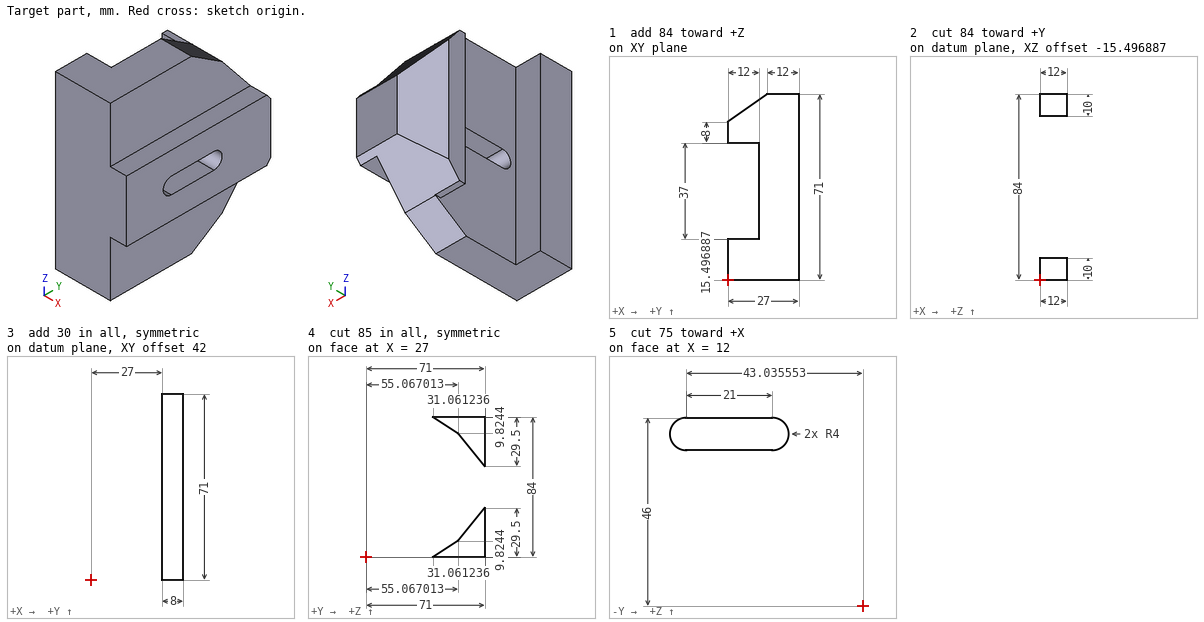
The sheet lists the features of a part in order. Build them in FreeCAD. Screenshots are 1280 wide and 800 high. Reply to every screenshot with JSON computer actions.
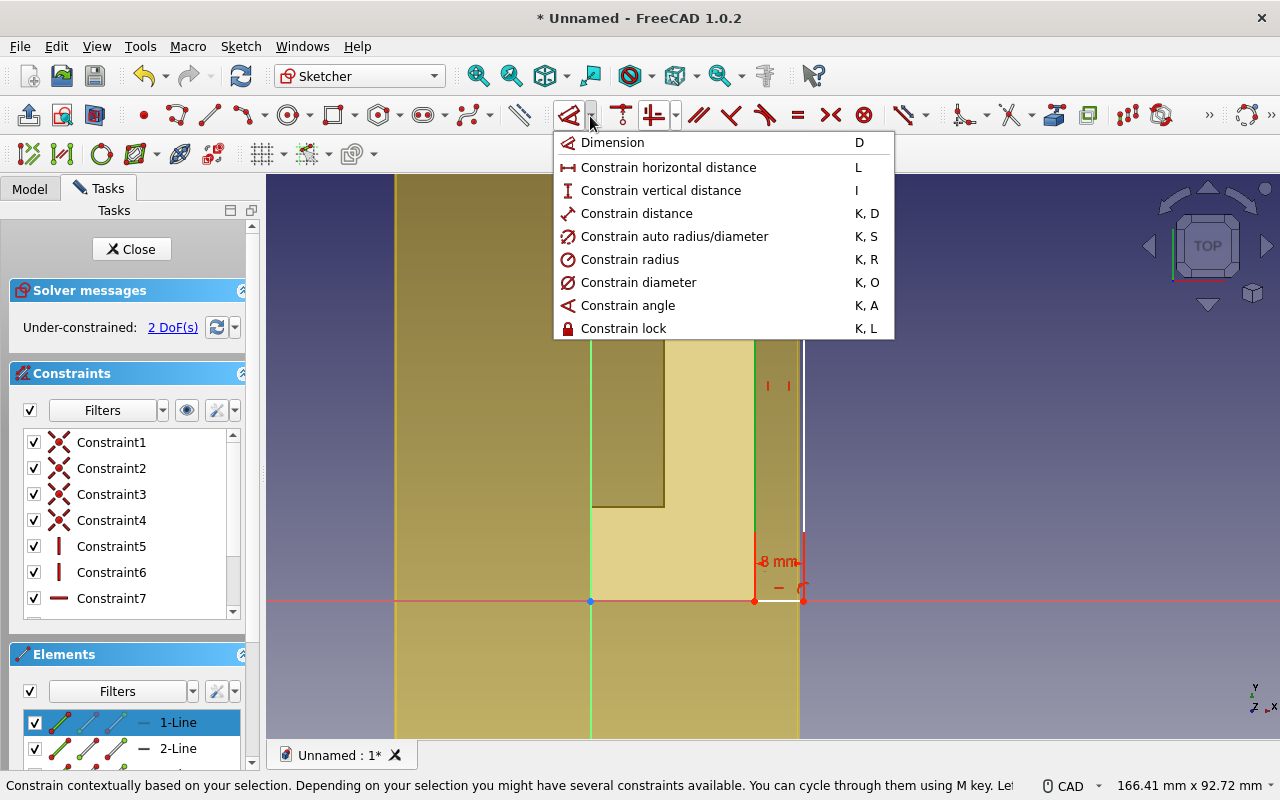
{"action": "left_click", "coordinate": [724, 190]}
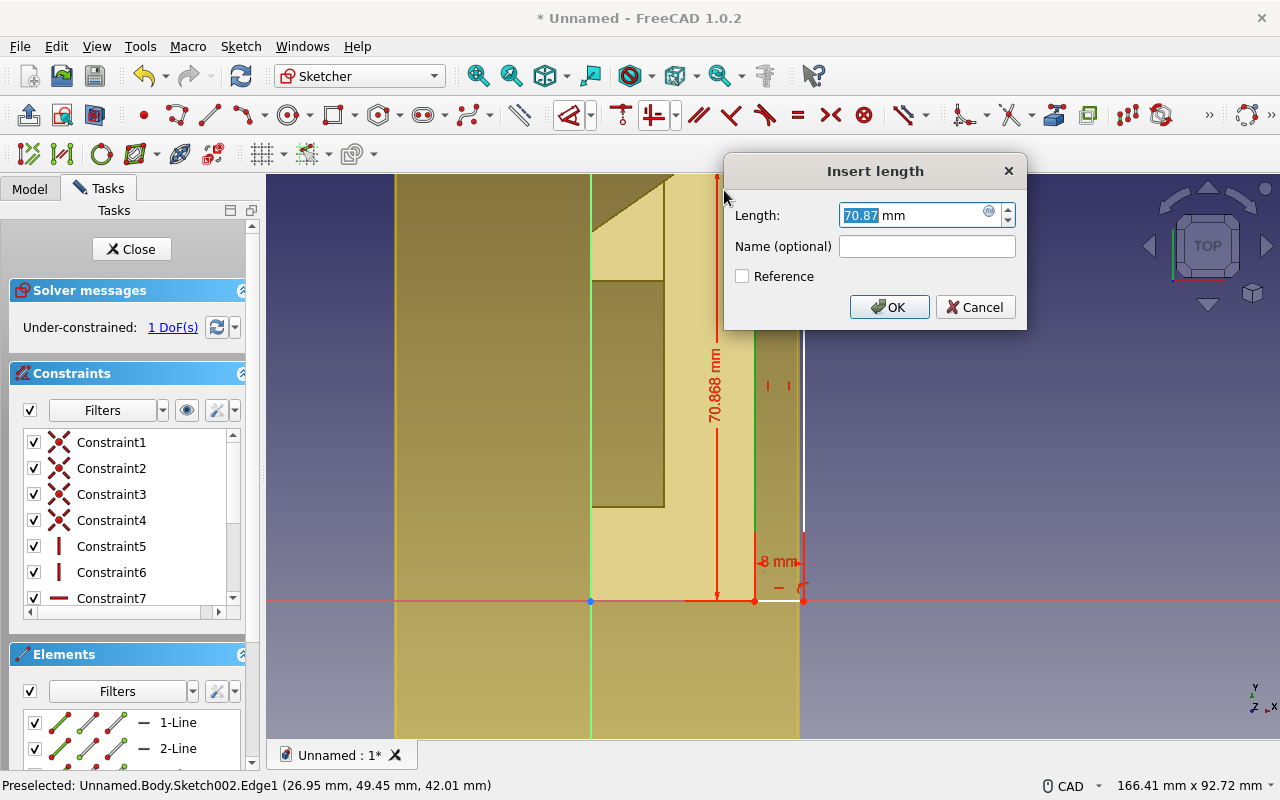
{"action": "type", "text": "71"}
{"action": "key", "text": "Return"}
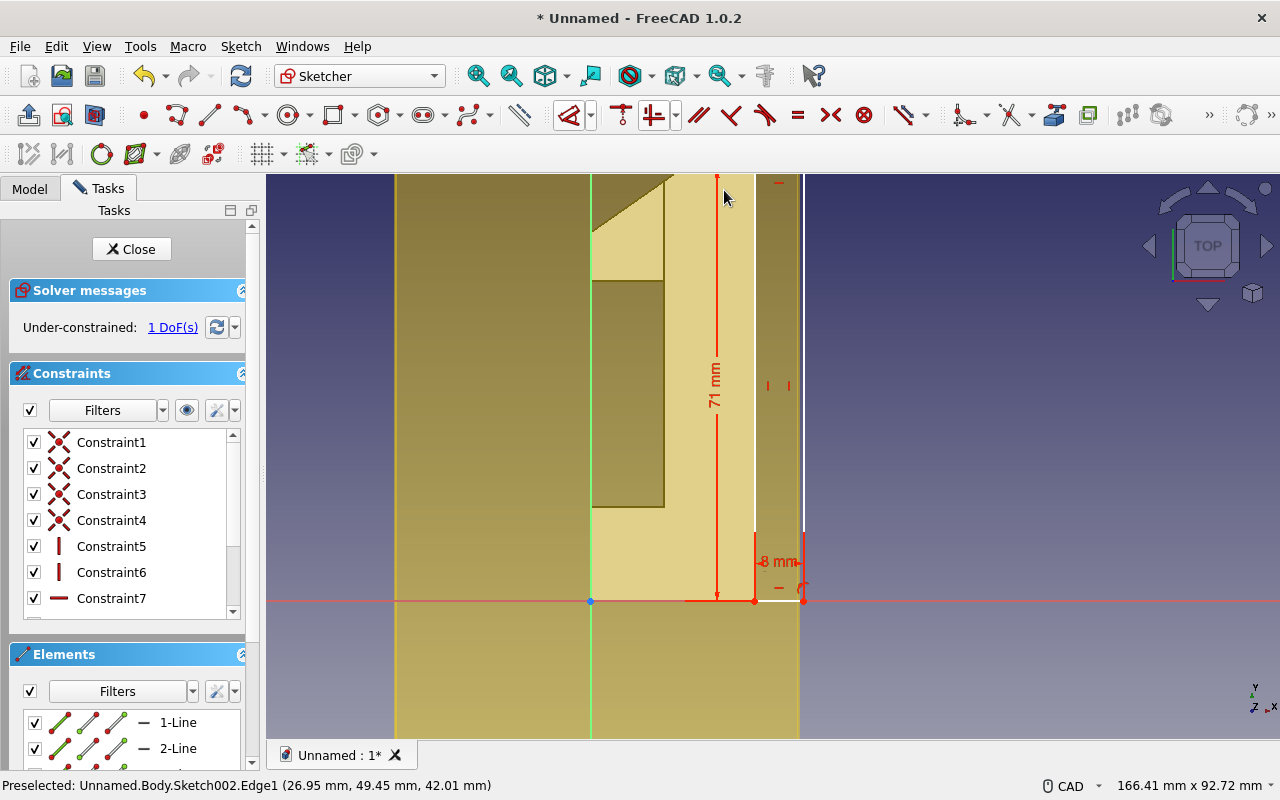
{"action": "scroll", "coordinate": [737, 711], "scroll_direction": "down", "scroll_amount": 1}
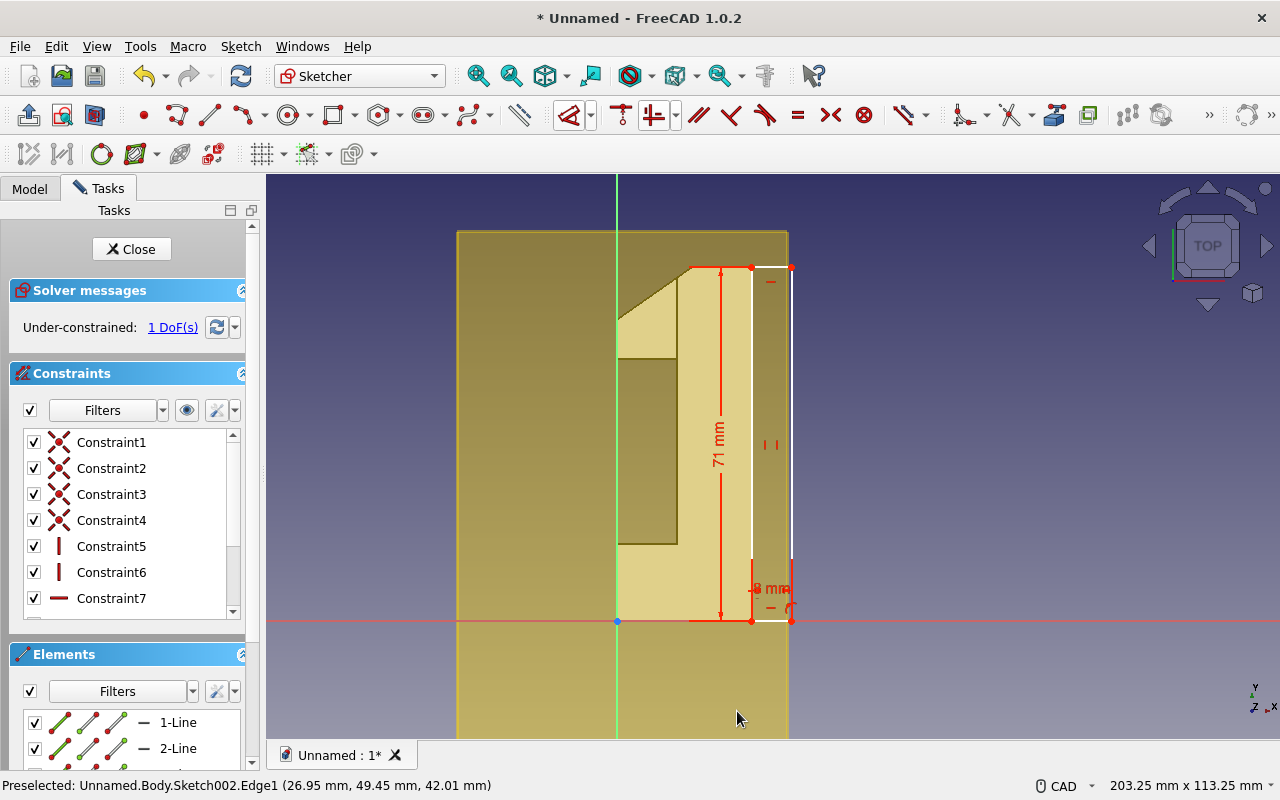
{"action": "left_click", "coordinate": [752, 267]}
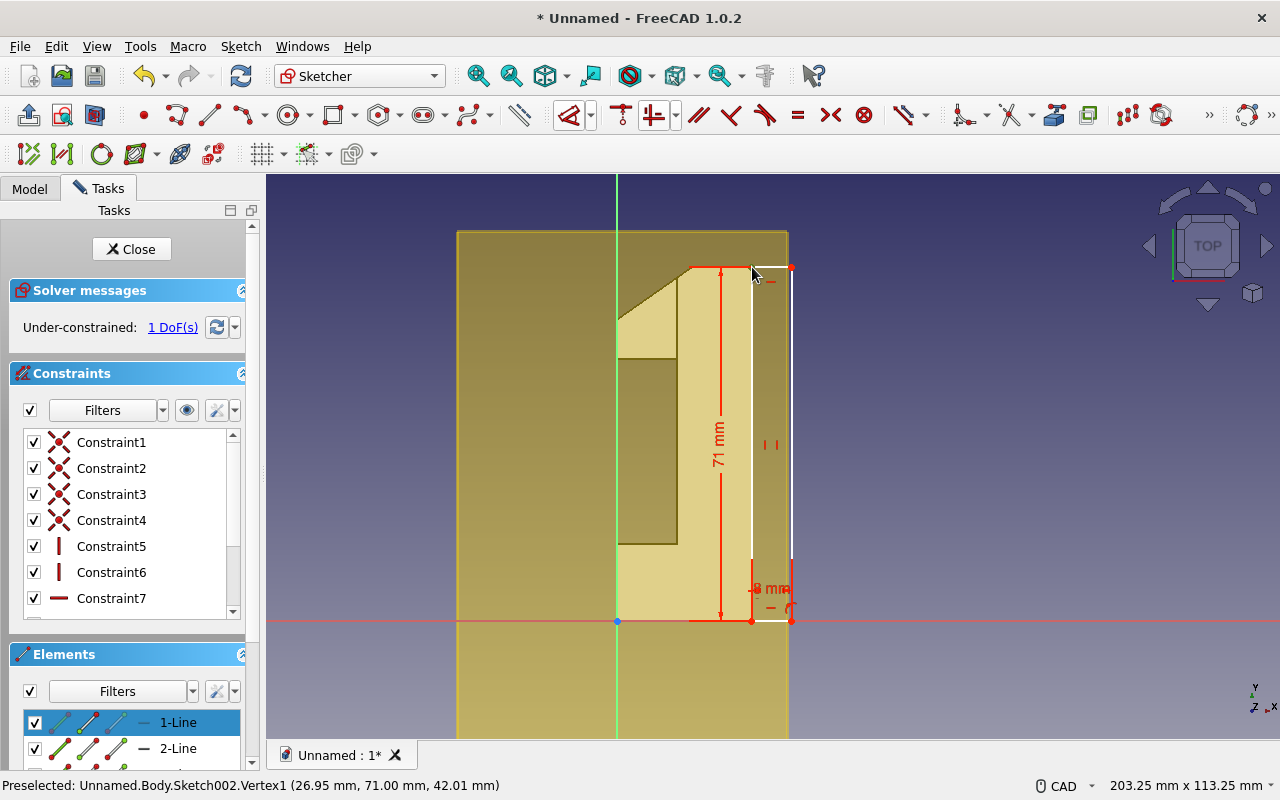
{"action": "left_click", "coordinate": [590, 116]}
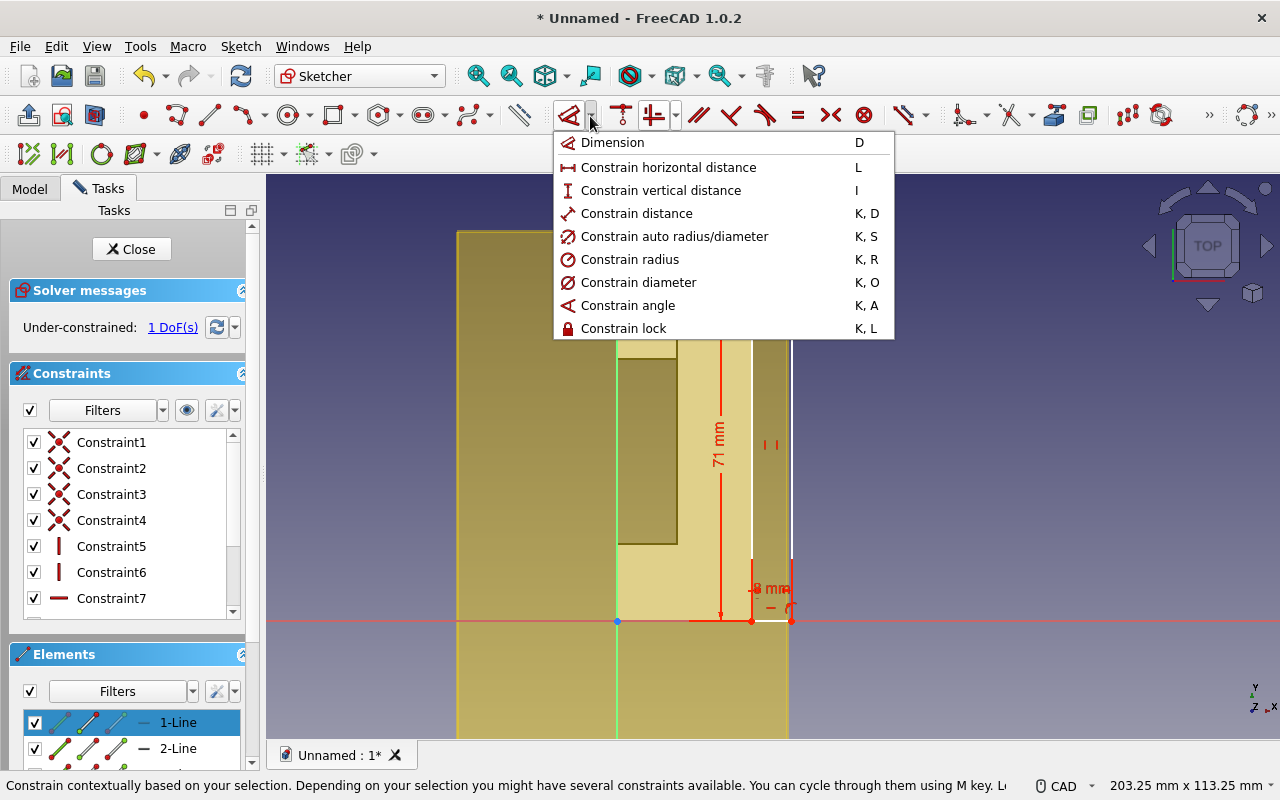
{"action": "left_click", "coordinate": [724, 168]}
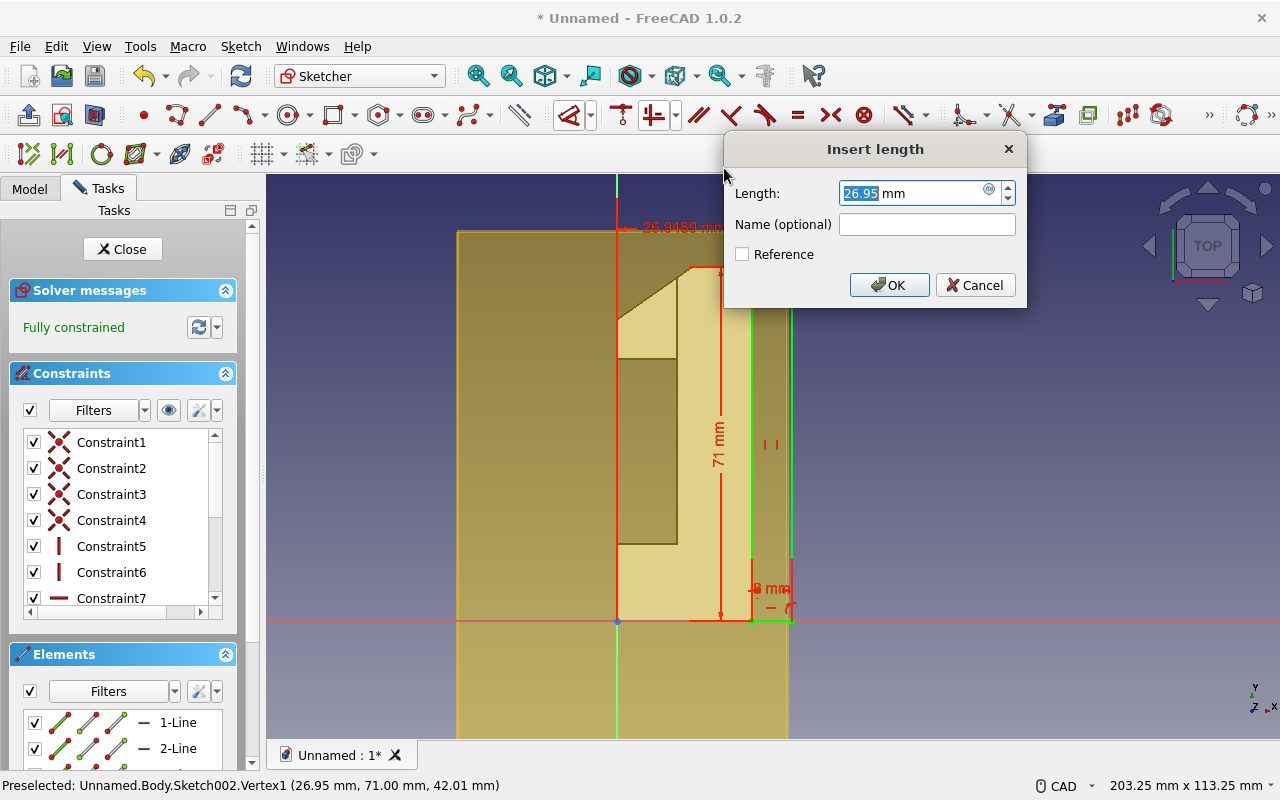
{"action": "type", "text": "27"}
{"action": "key", "text": "Return"}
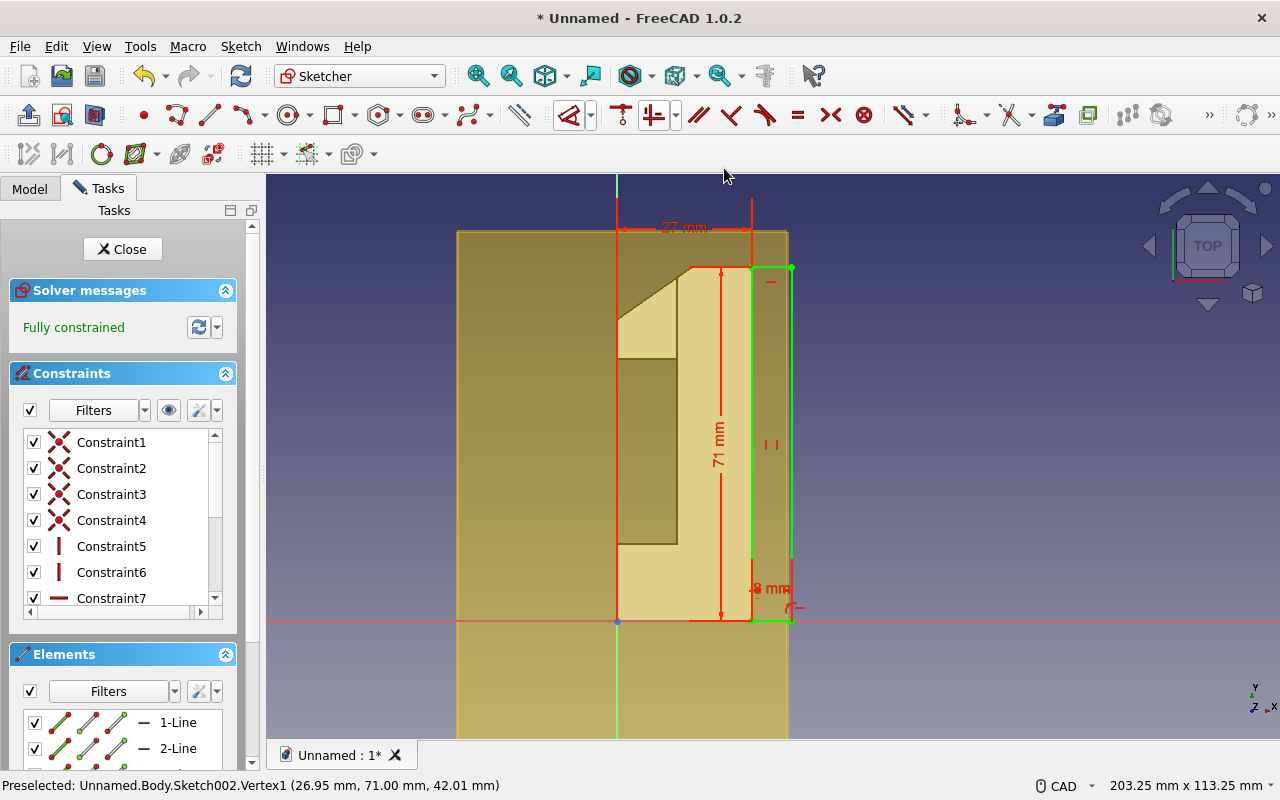
{"action": "left_click", "coordinate": [123, 249]}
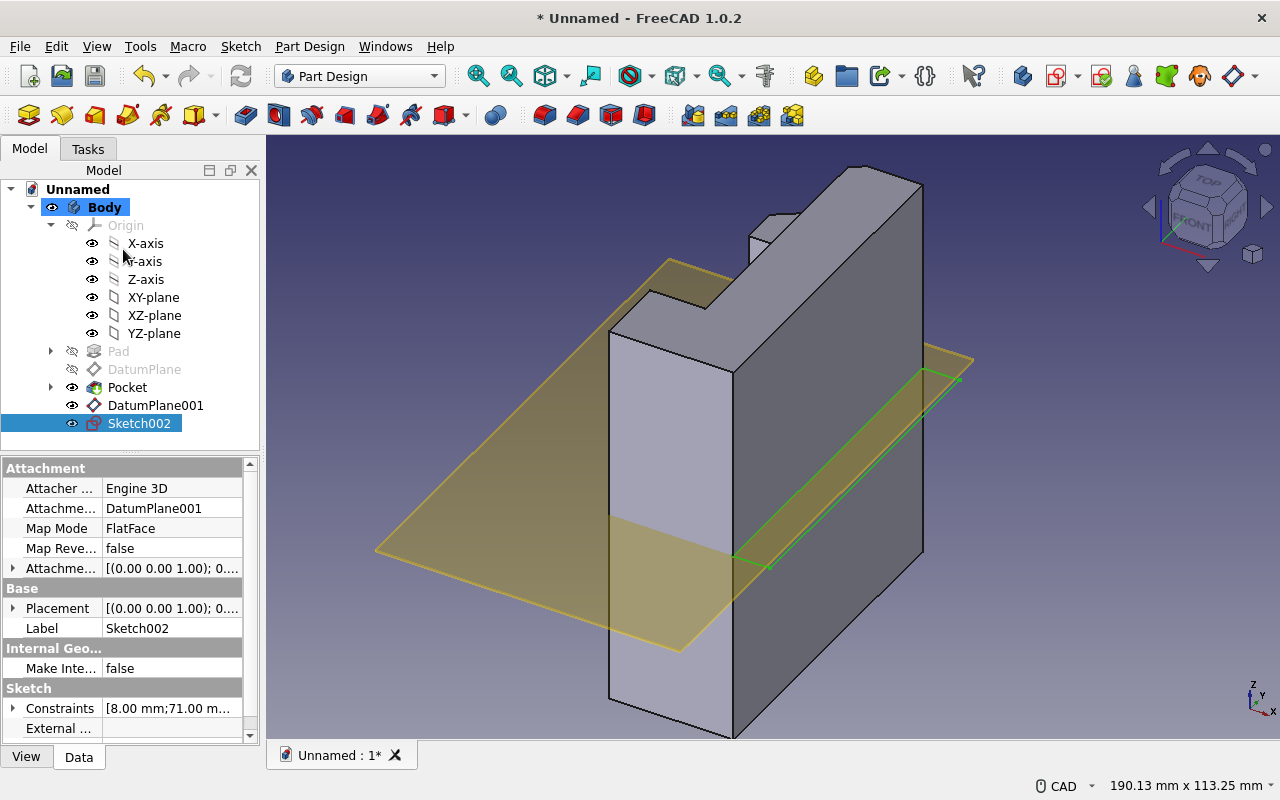
{"action": "left_click", "coordinate": [29, 116]}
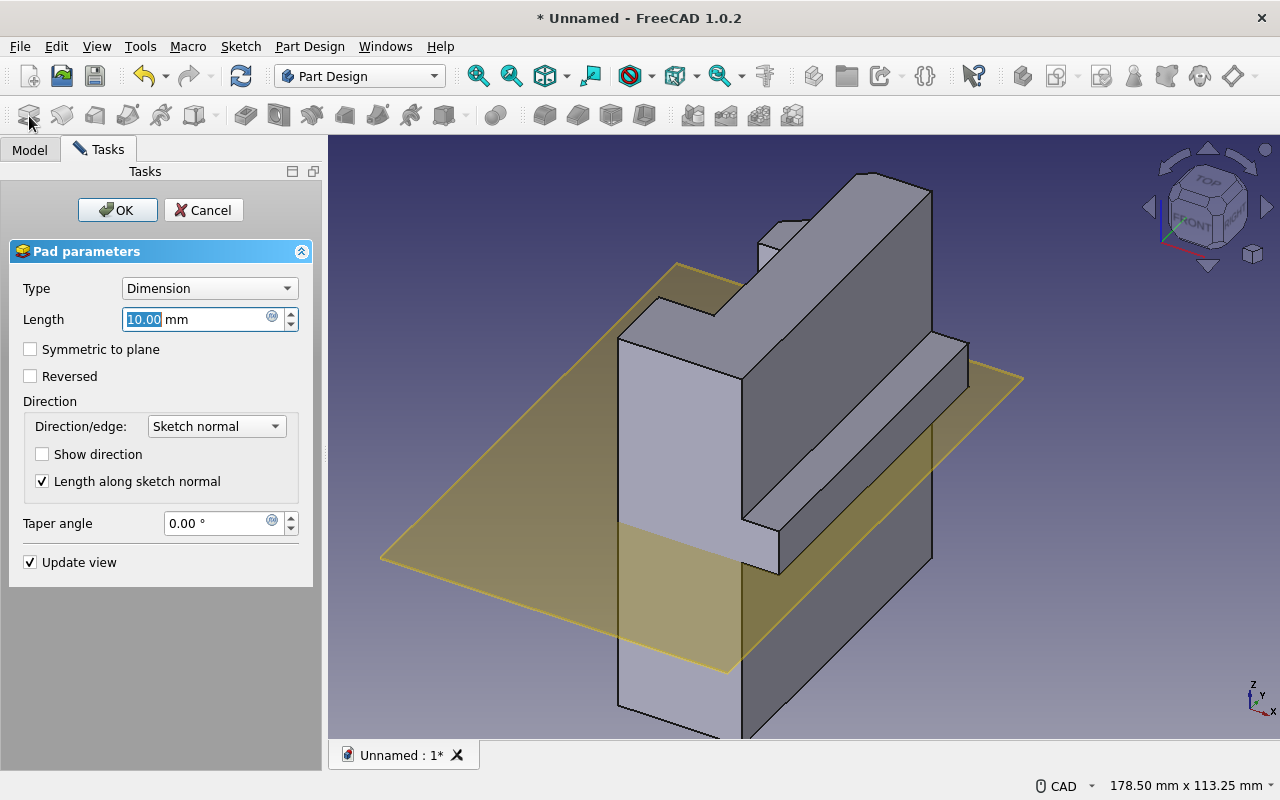
{"action": "type", "text": "30"}
{"action": "key", "text": "Tab"}